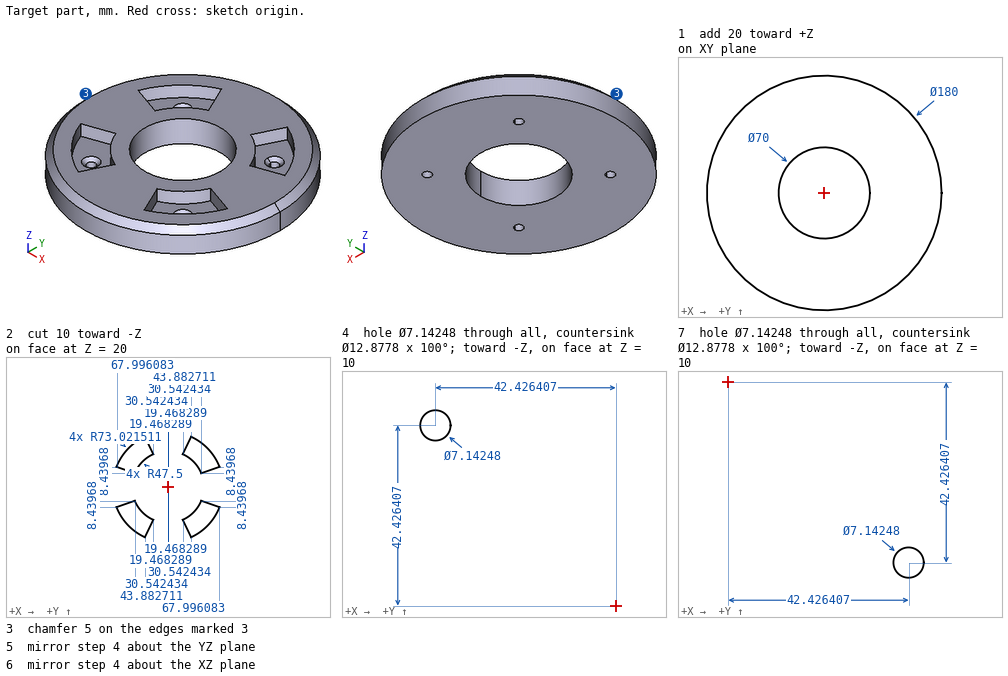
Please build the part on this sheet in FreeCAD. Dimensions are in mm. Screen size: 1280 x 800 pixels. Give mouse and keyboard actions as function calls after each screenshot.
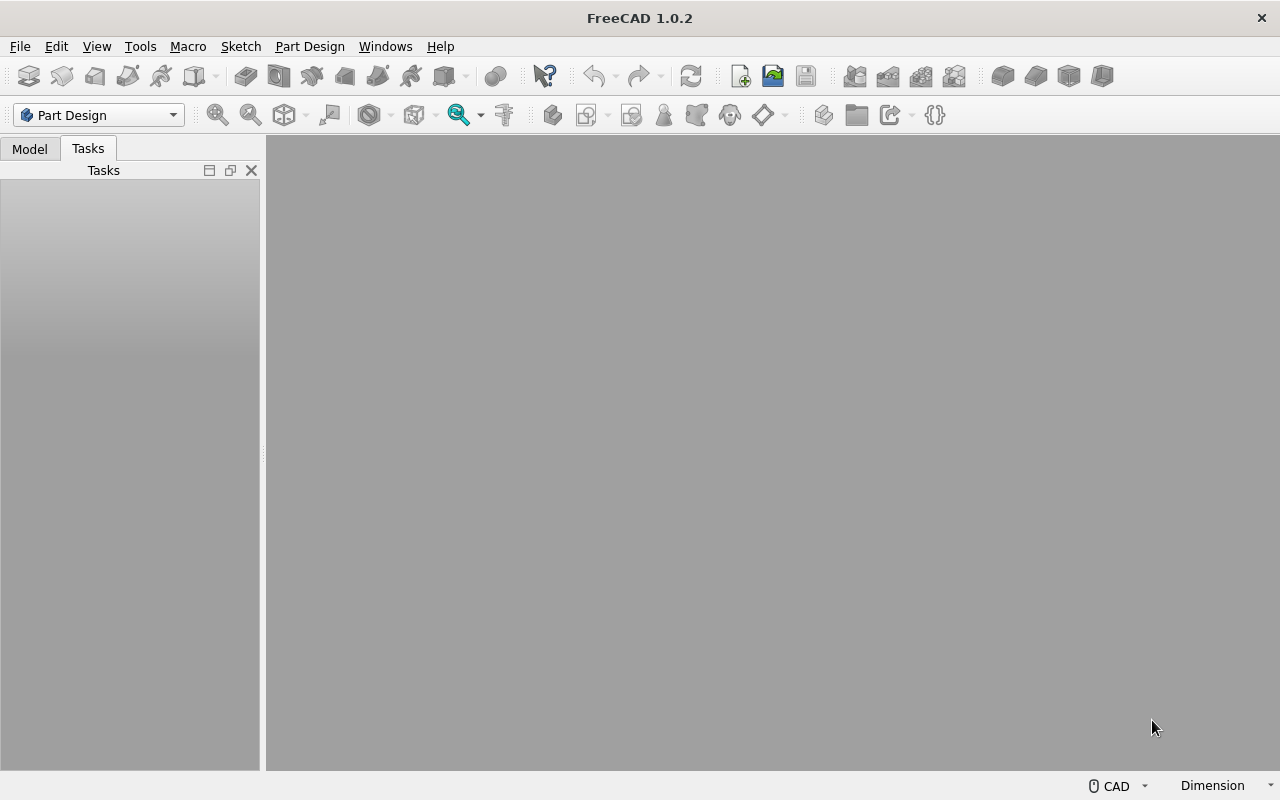
click(740, 76)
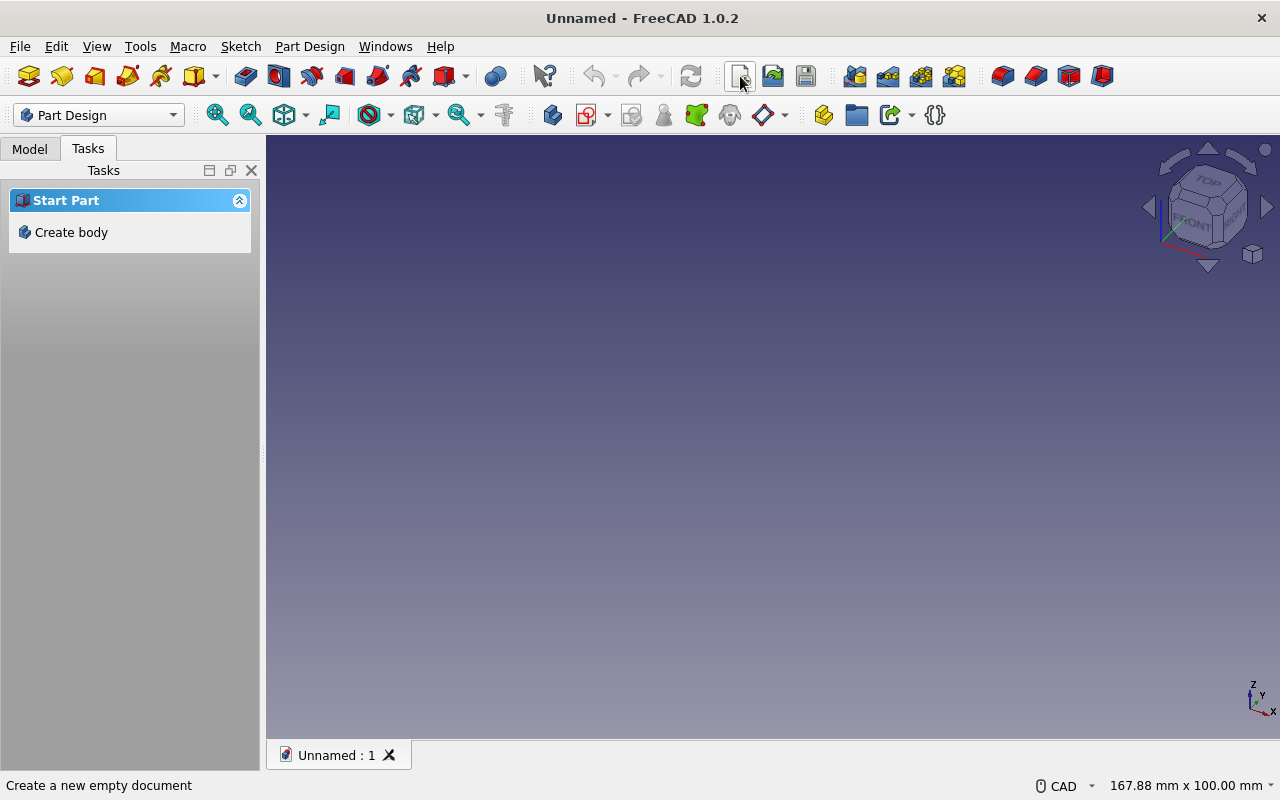
click(586, 116)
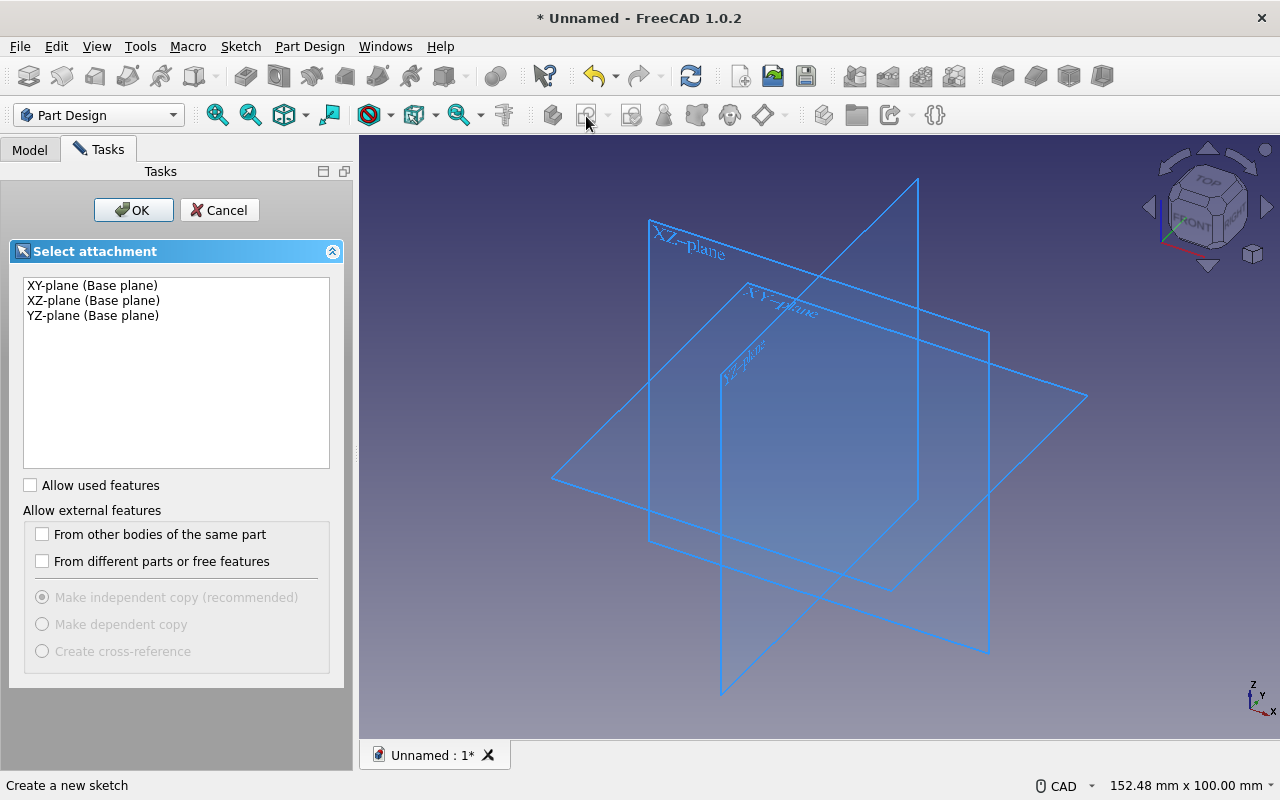
click(84, 286)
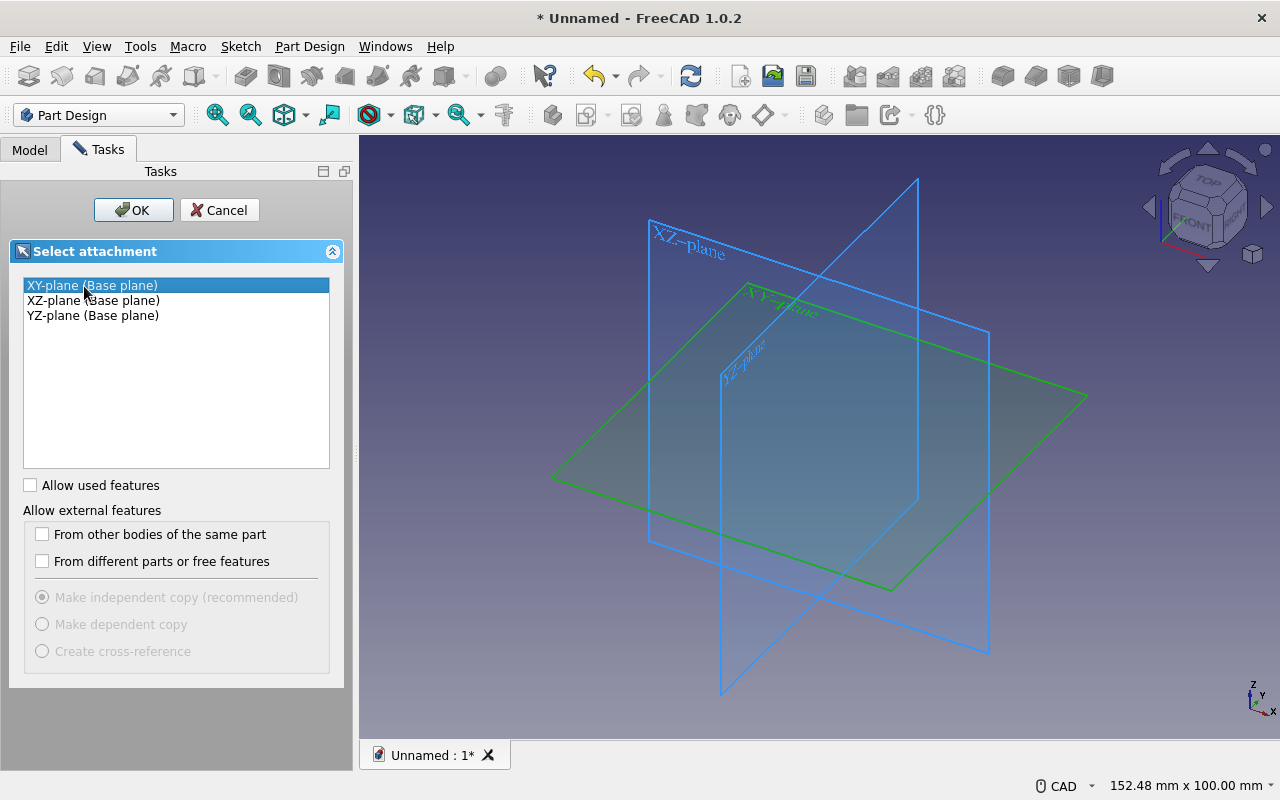
click(134, 210)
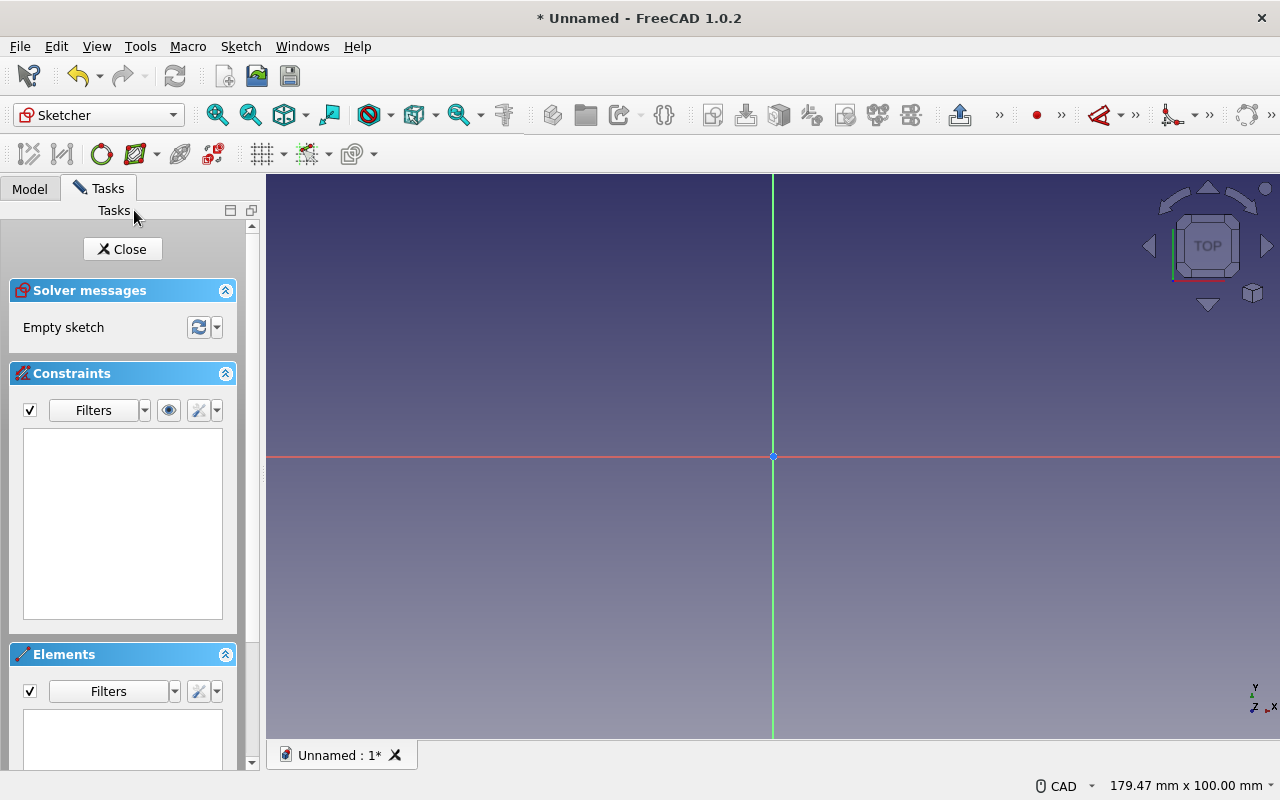
scroll(665, 456, down, 5)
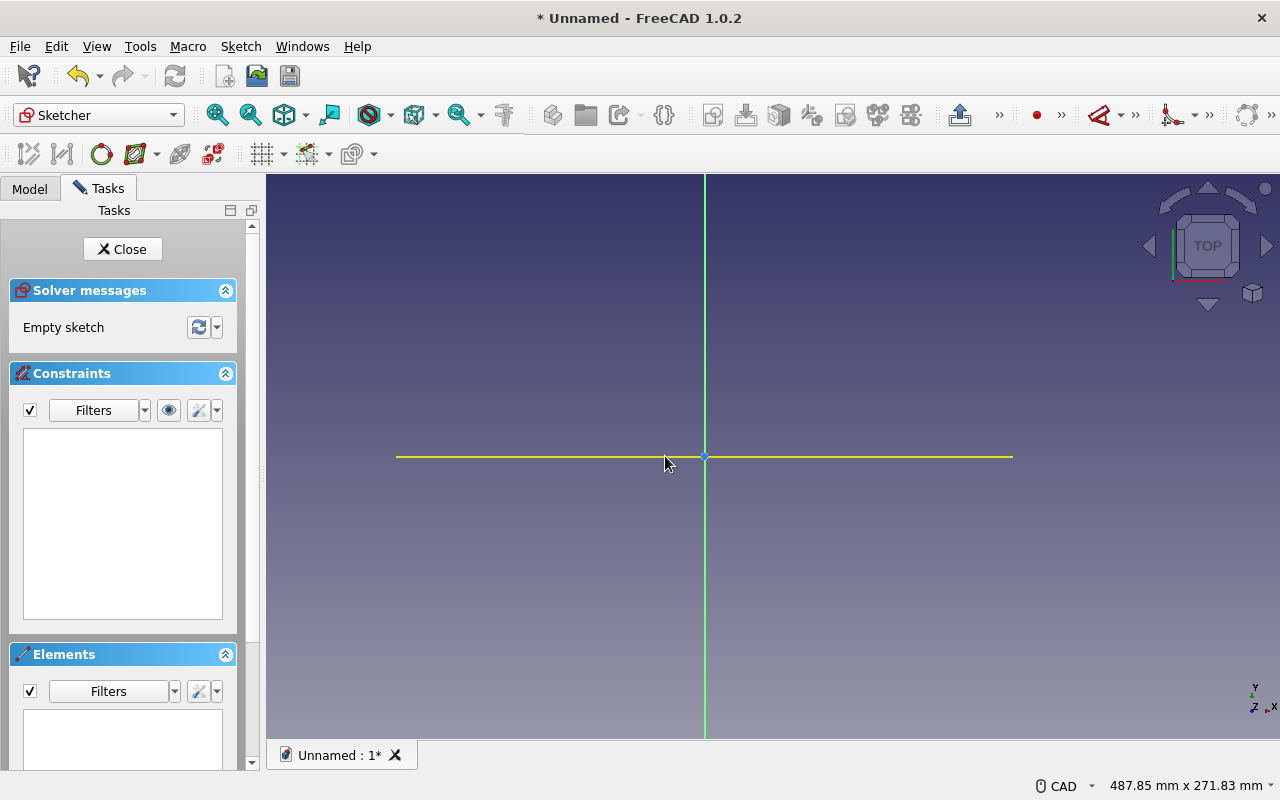
key(g)
key(c)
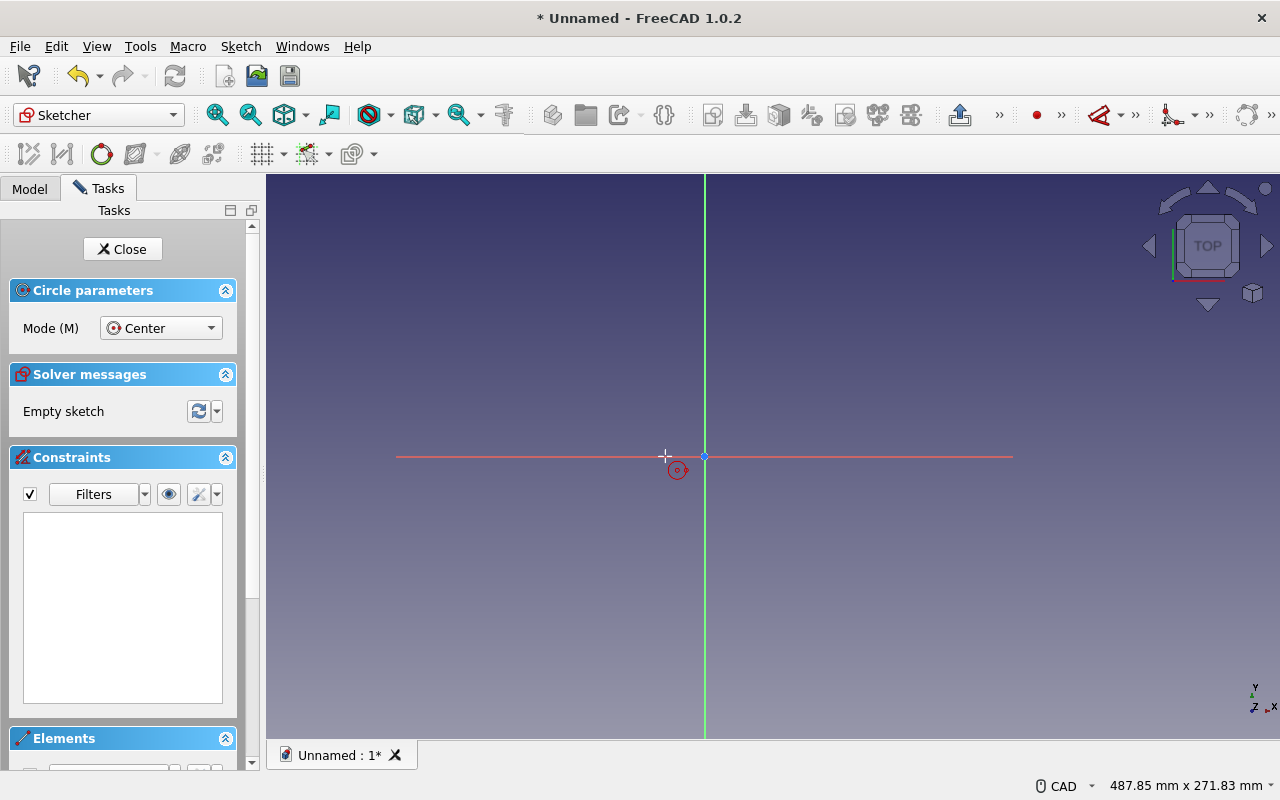
click(705, 456)
move(837, 324)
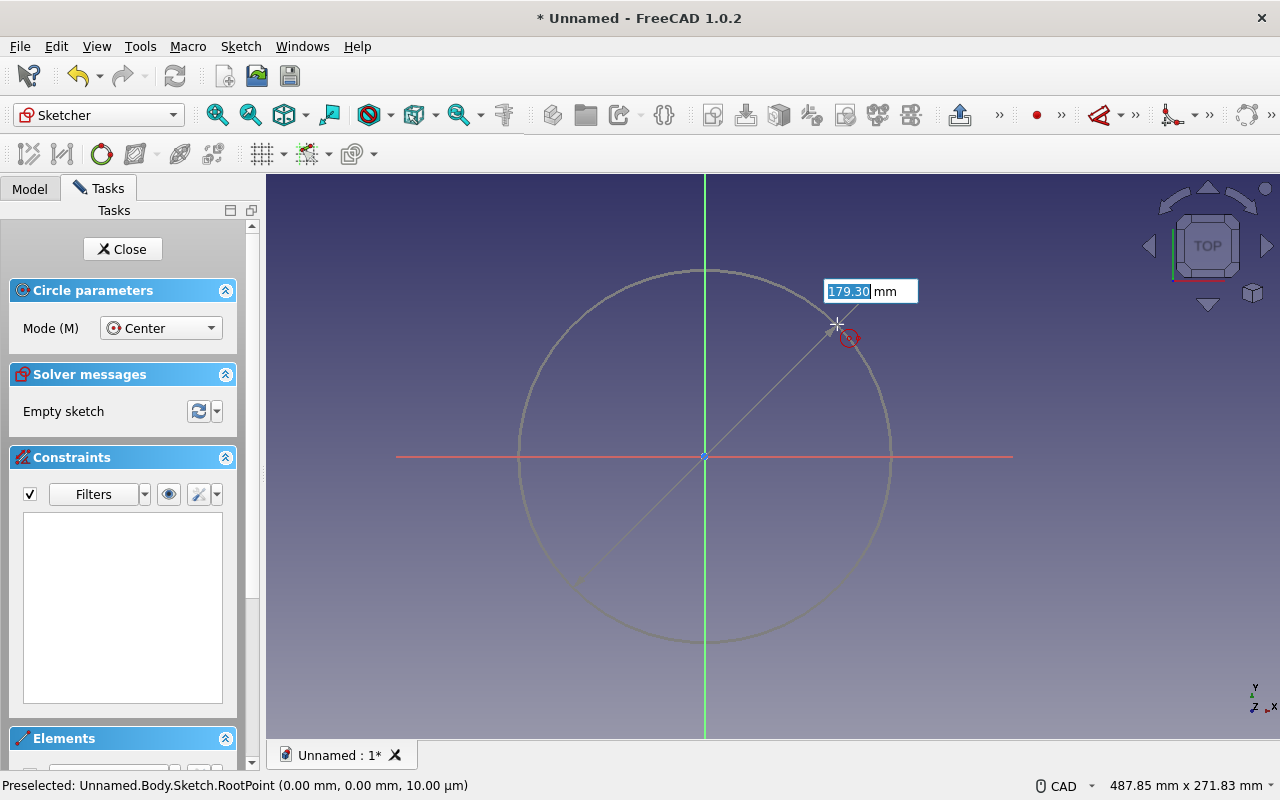
text(180)
key(Return)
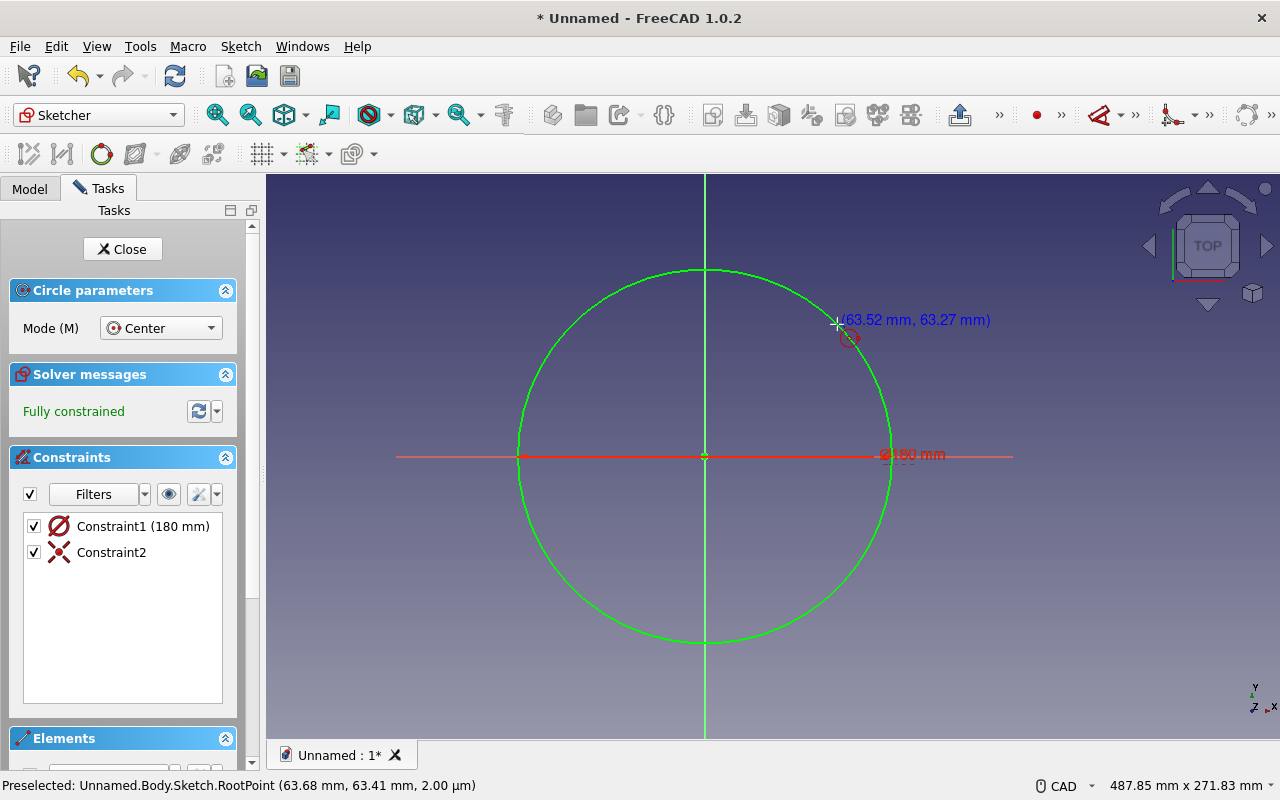
click(705, 456)
move(756, 405)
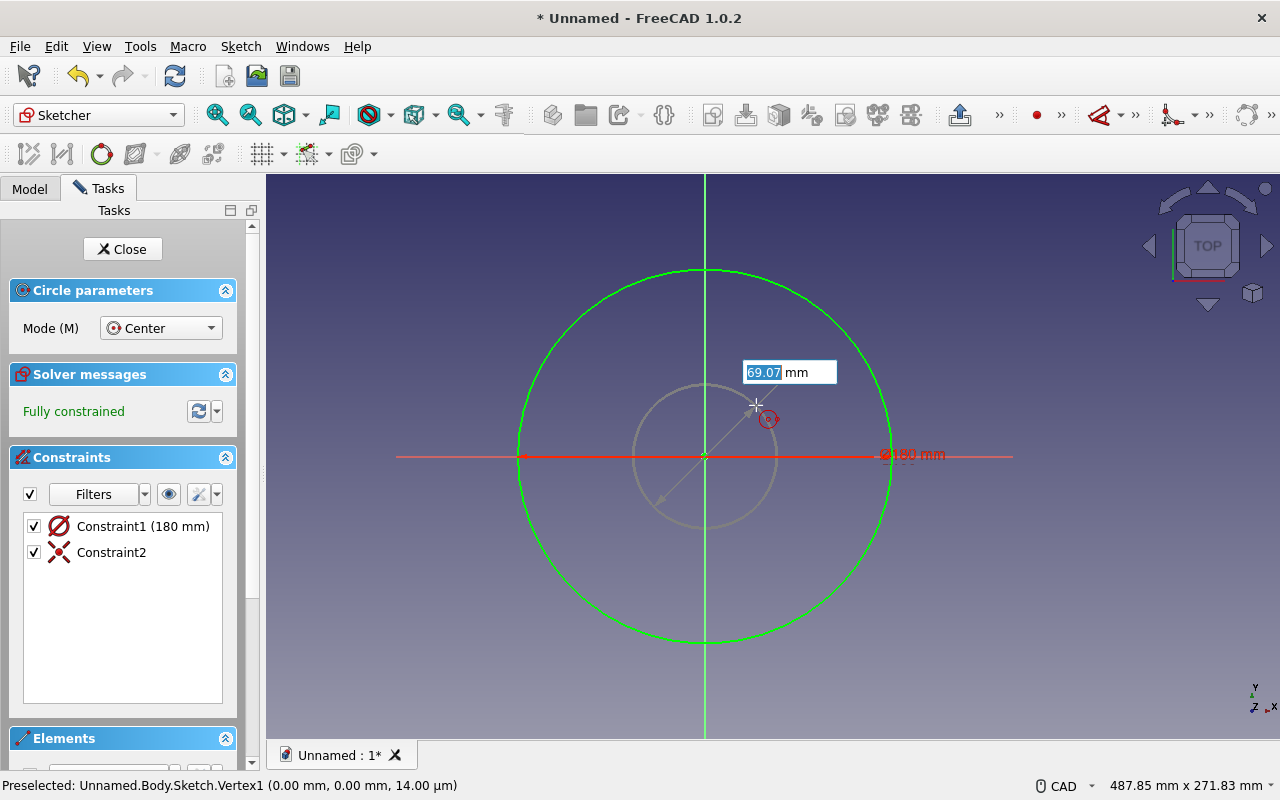
text(70)
key(Return)
key(Escape)